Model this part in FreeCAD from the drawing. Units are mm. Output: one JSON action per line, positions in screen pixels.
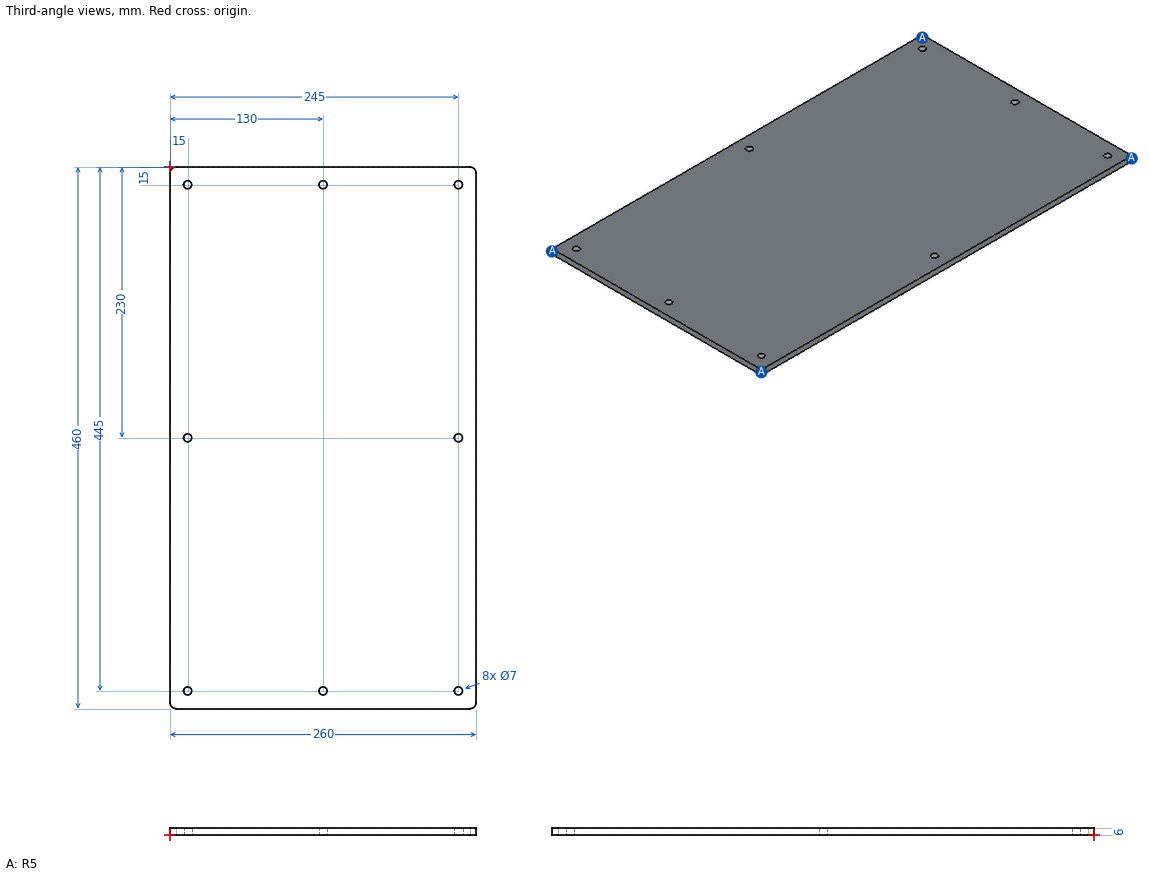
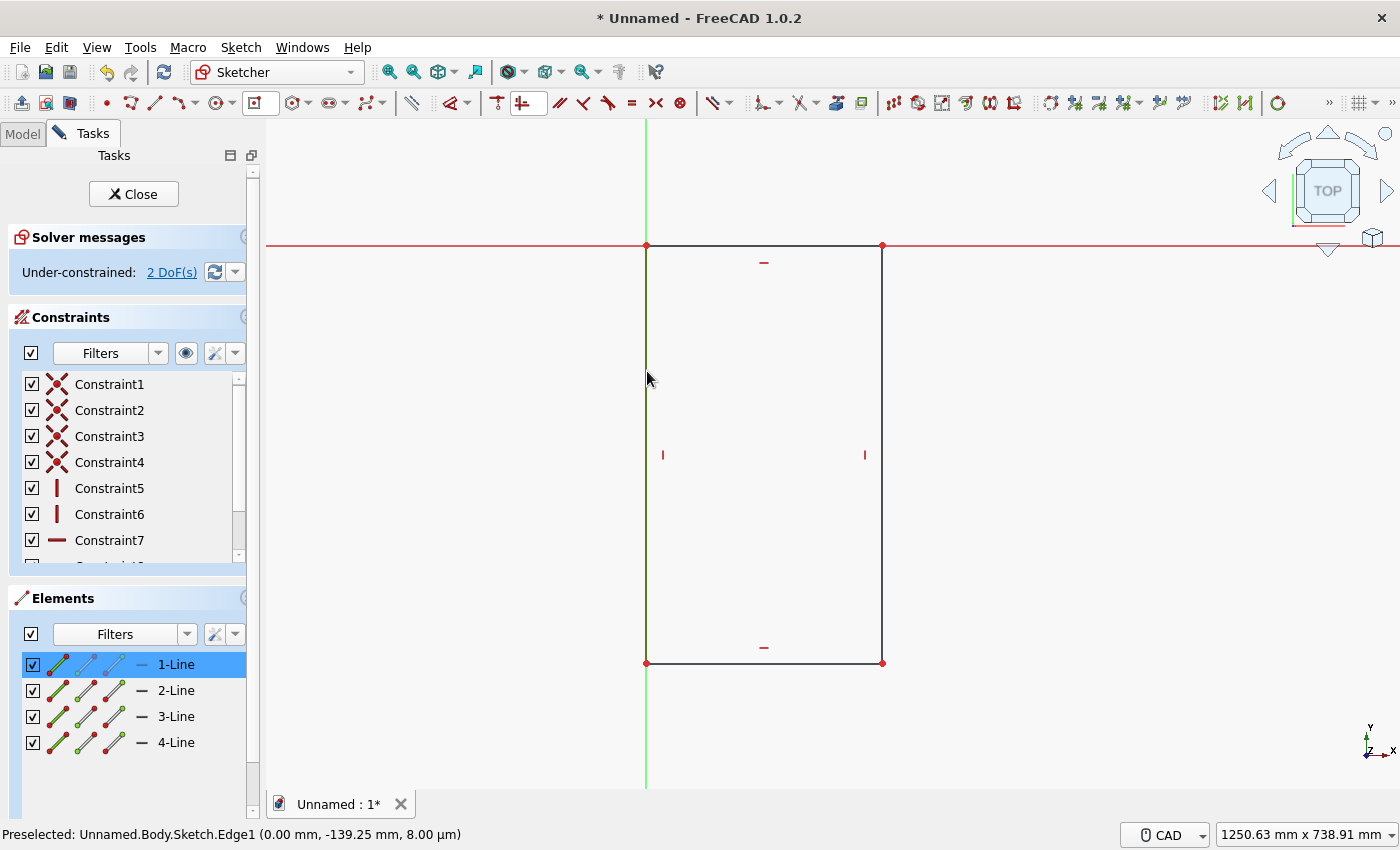
{"action": "key", "text": "i"}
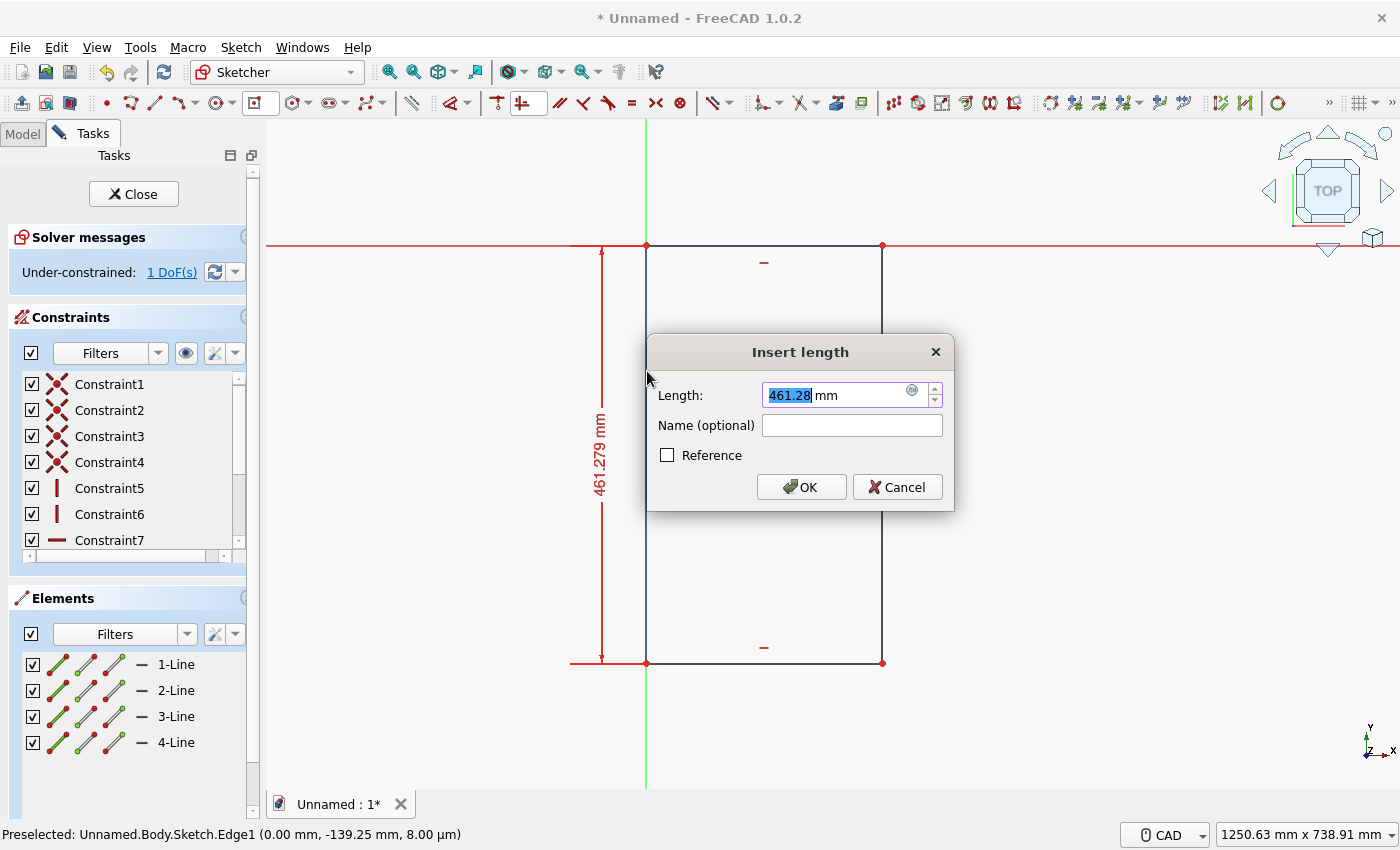
{"action": "type", "text": "460"}
{"action": "key", "text": "Return"}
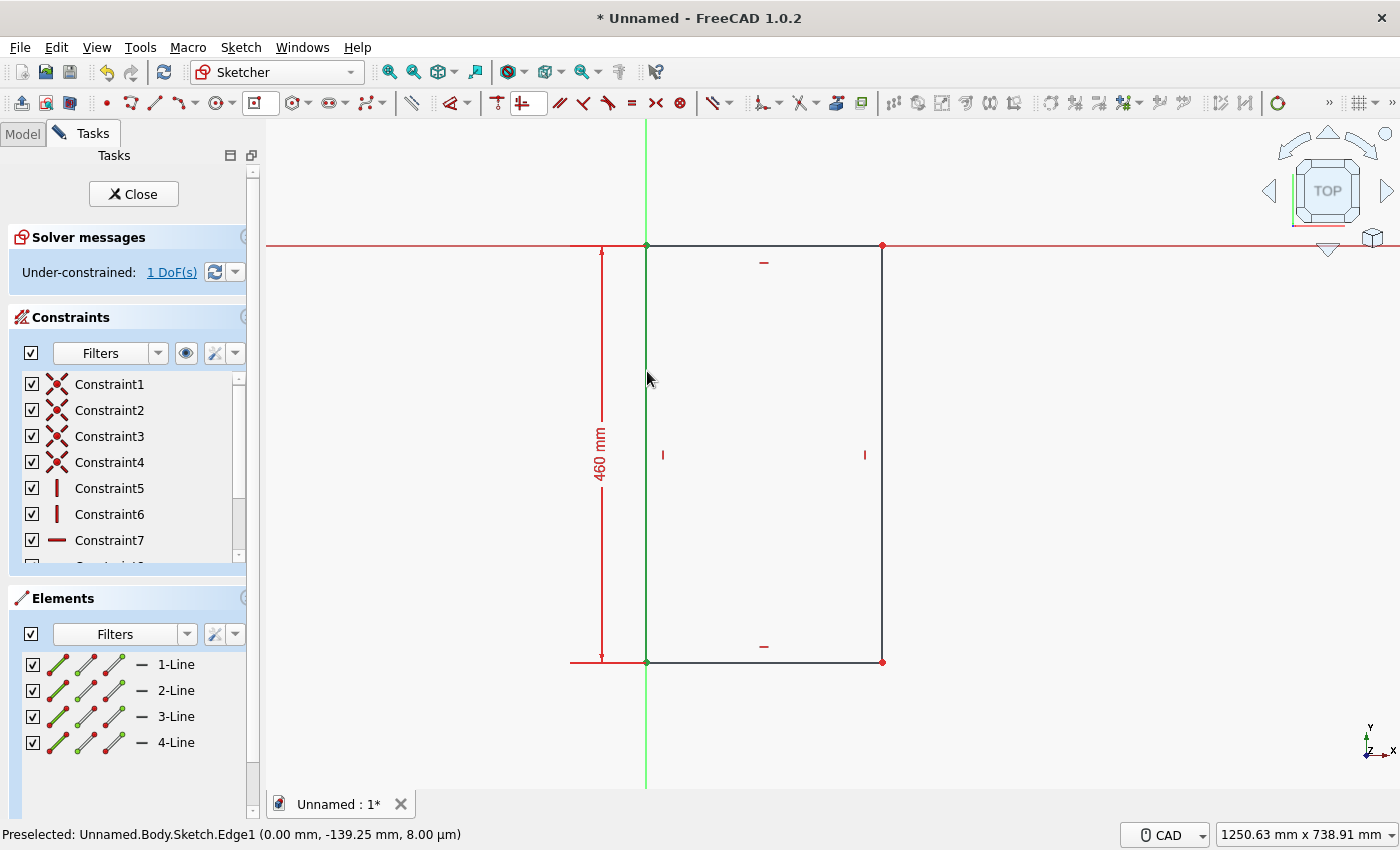
{"action": "left_click", "coordinate": [717, 663]}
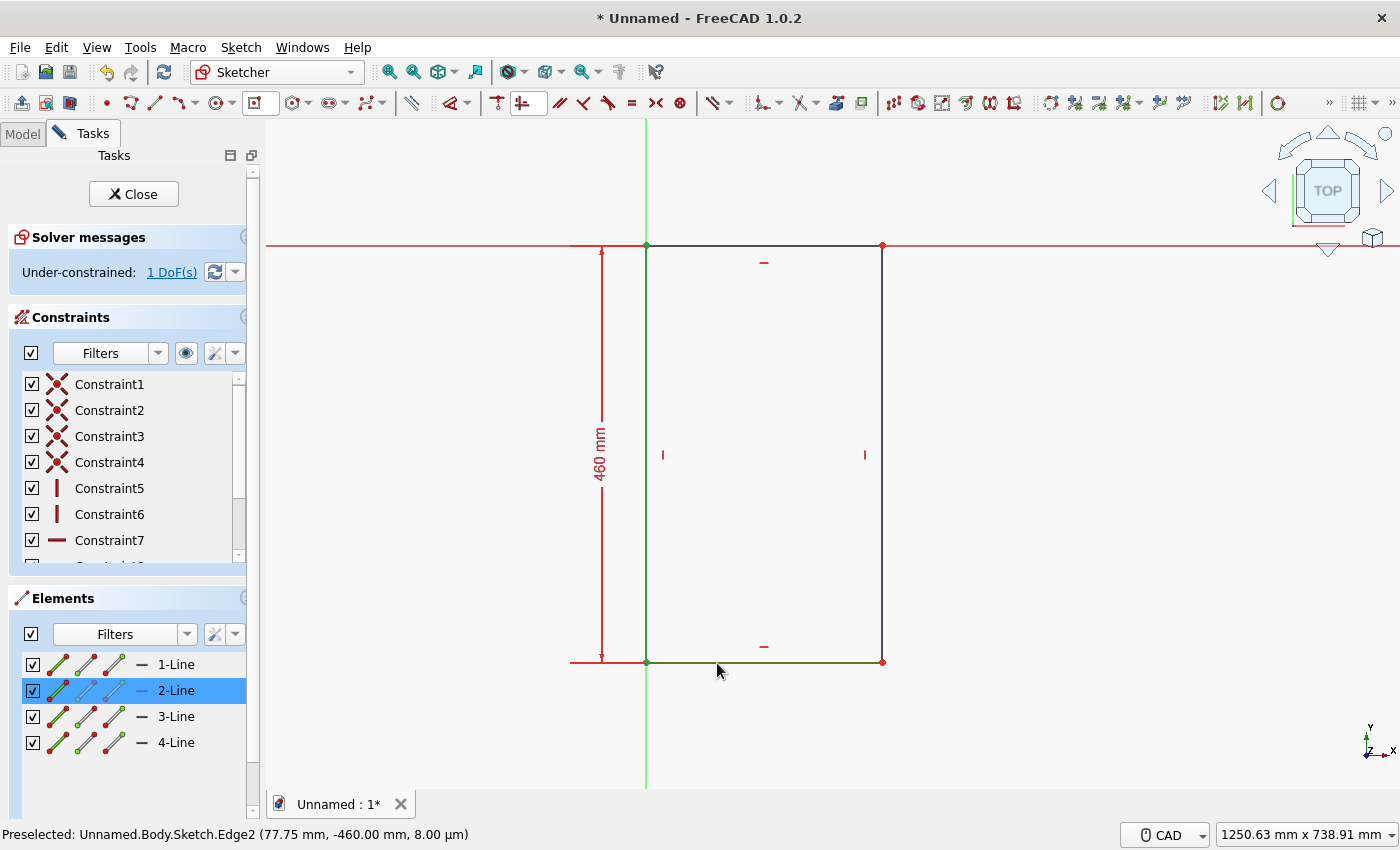
{"action": "key", "text": "l"}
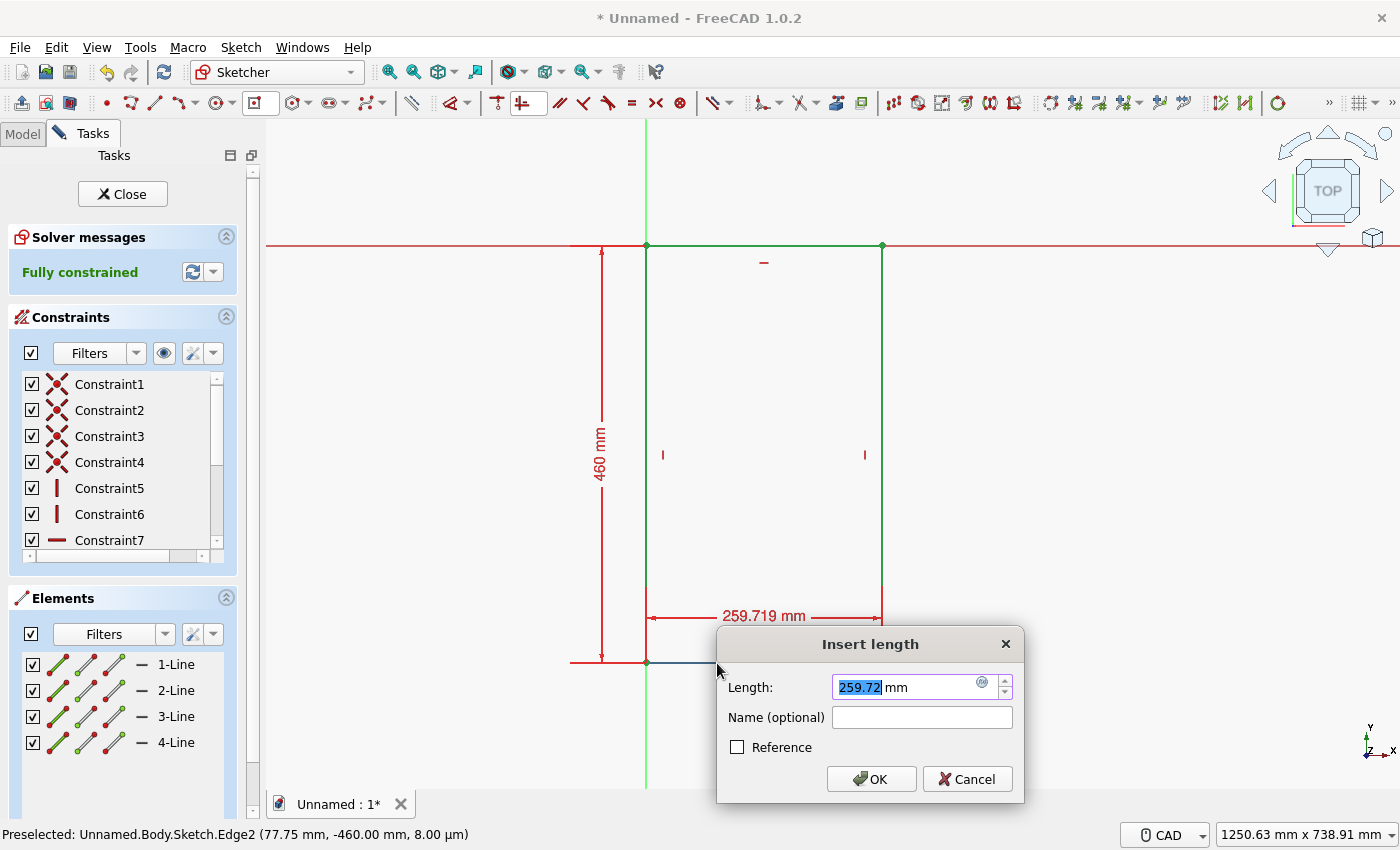
{"action": "type", "text": "260"}
{"action": "key", "text": "Return"}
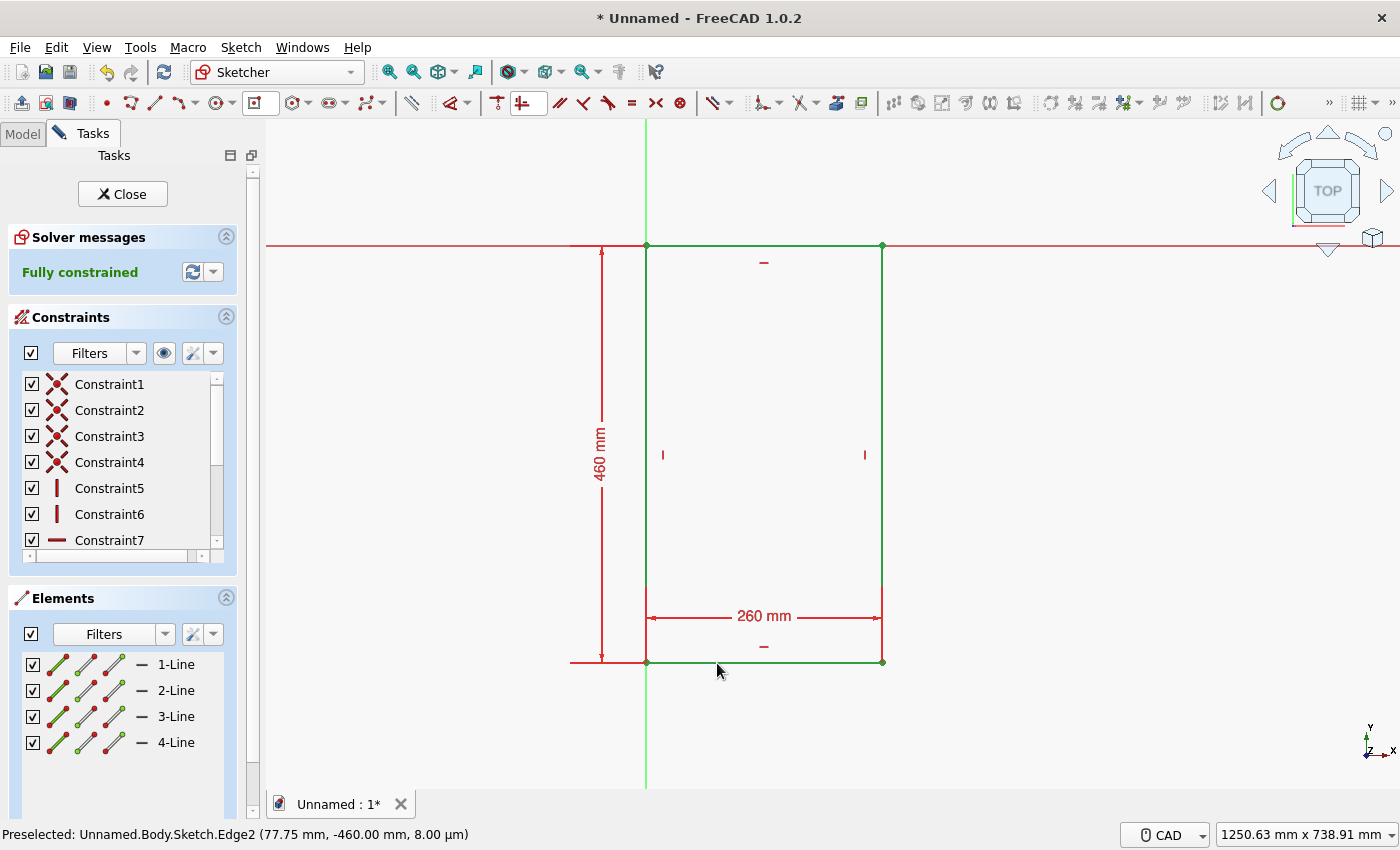
{"action": "left_click", "coordinate": [123, 194]}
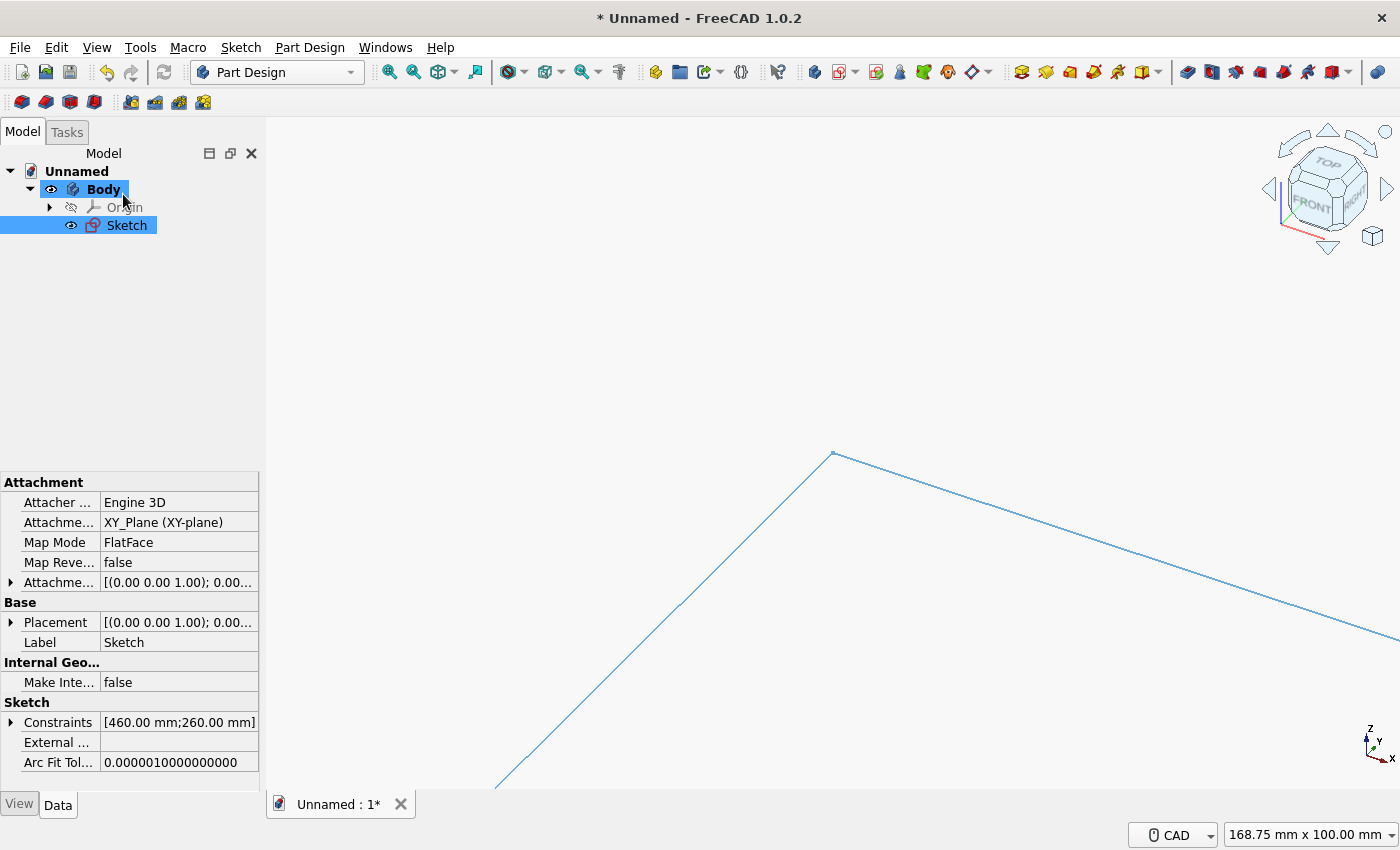
{"action": "left_click", "coordinate": [1022, 72]}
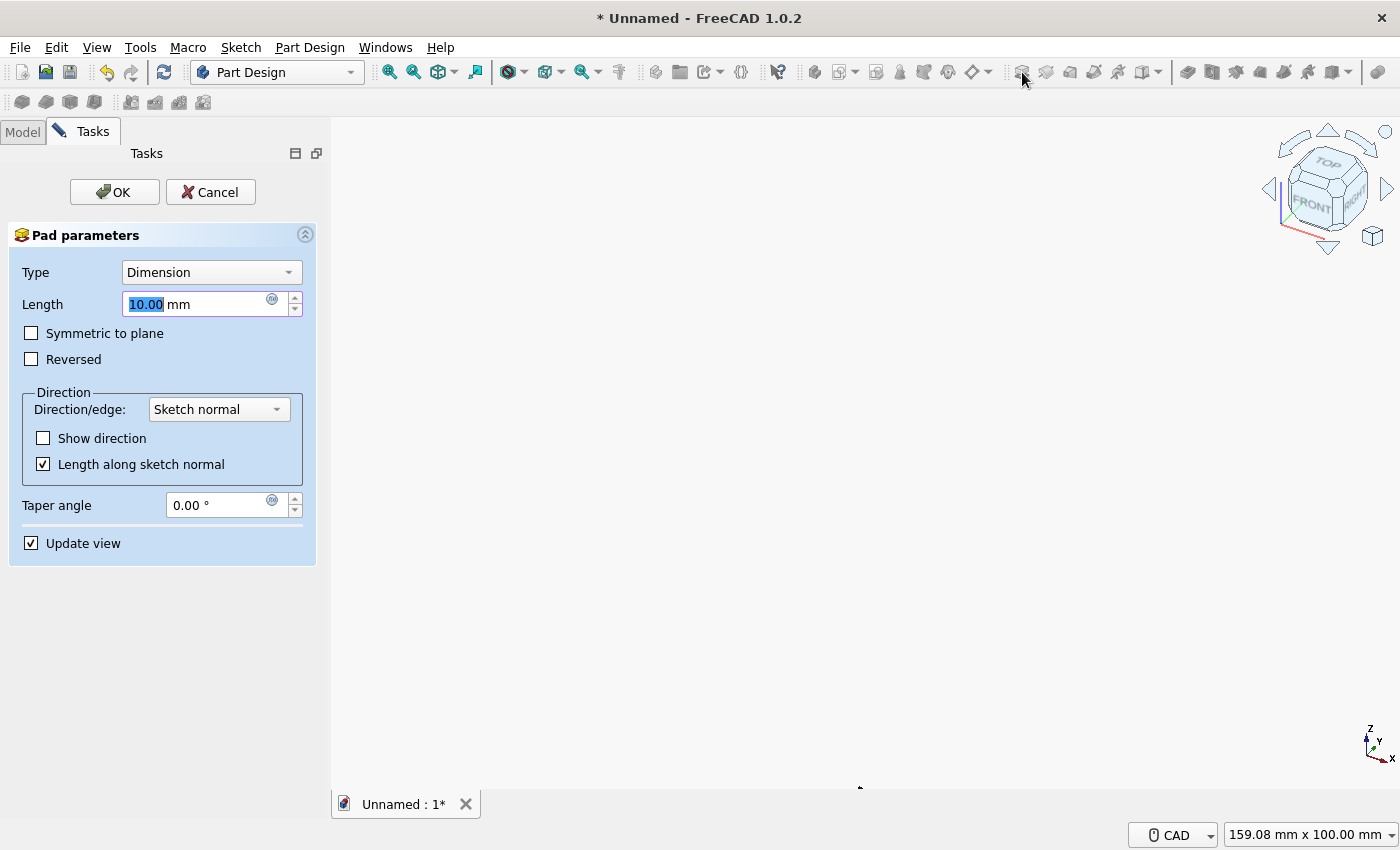
{"action": "type", "text": "6"}
{"action": "key", "text": "Tab"}